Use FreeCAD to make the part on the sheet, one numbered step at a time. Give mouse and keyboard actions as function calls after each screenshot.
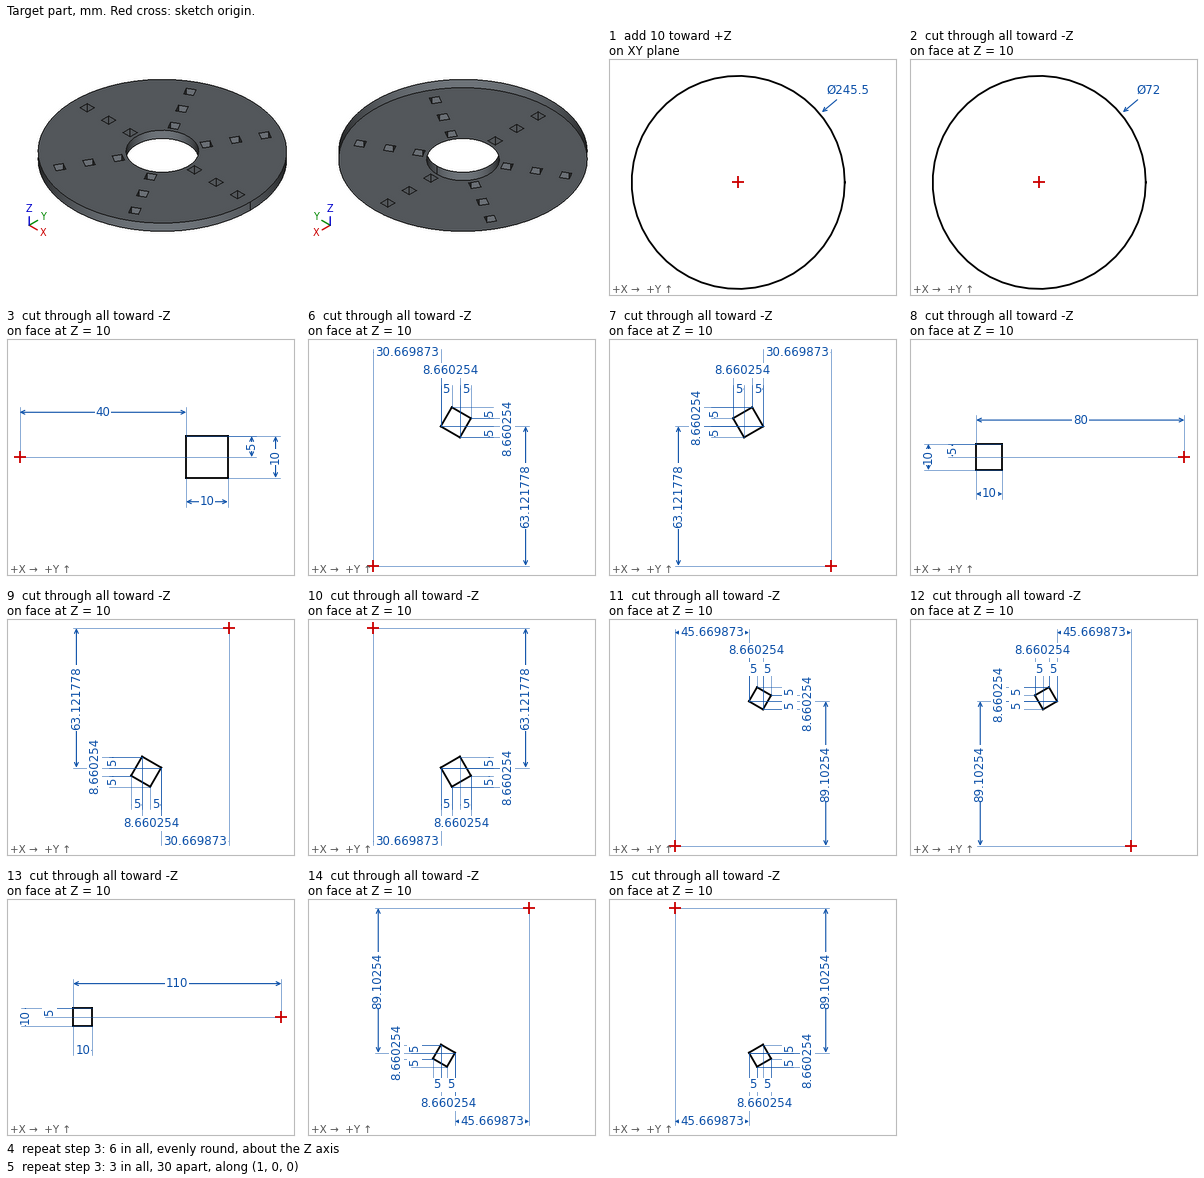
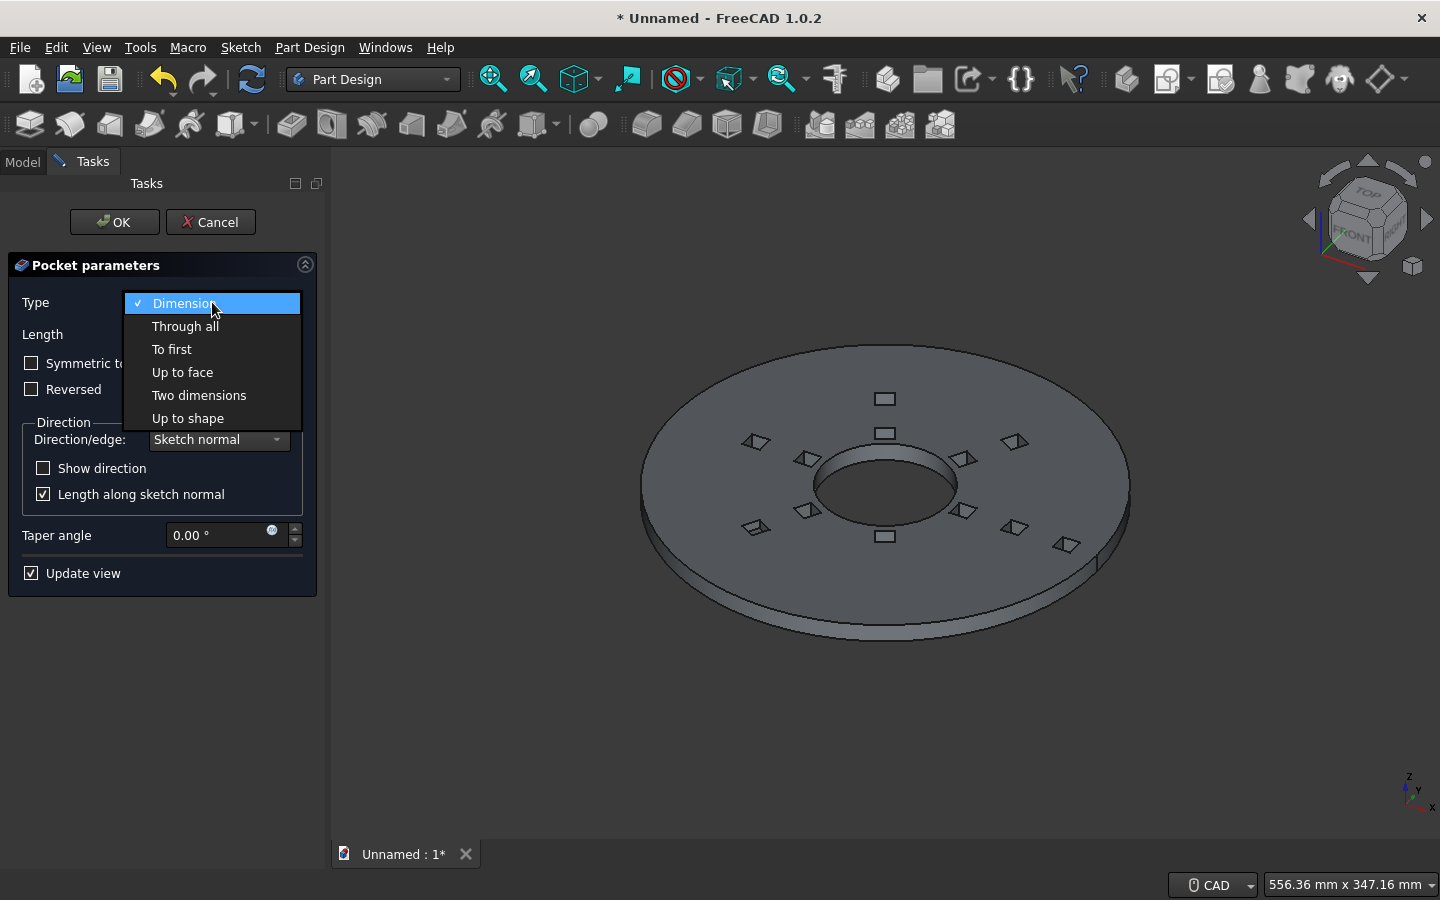
click(212, 326)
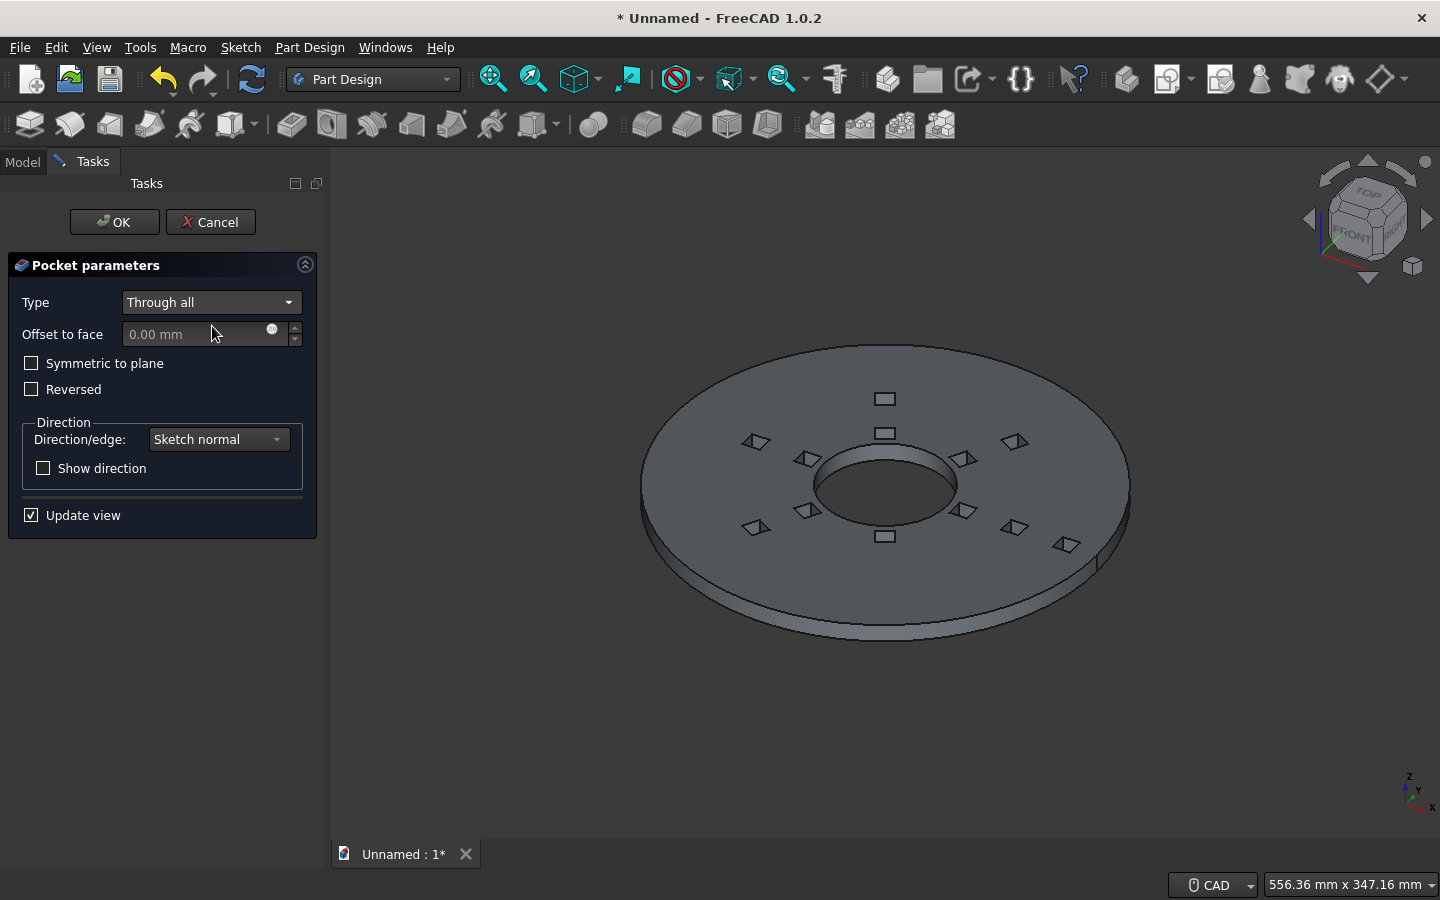
click(115, 222)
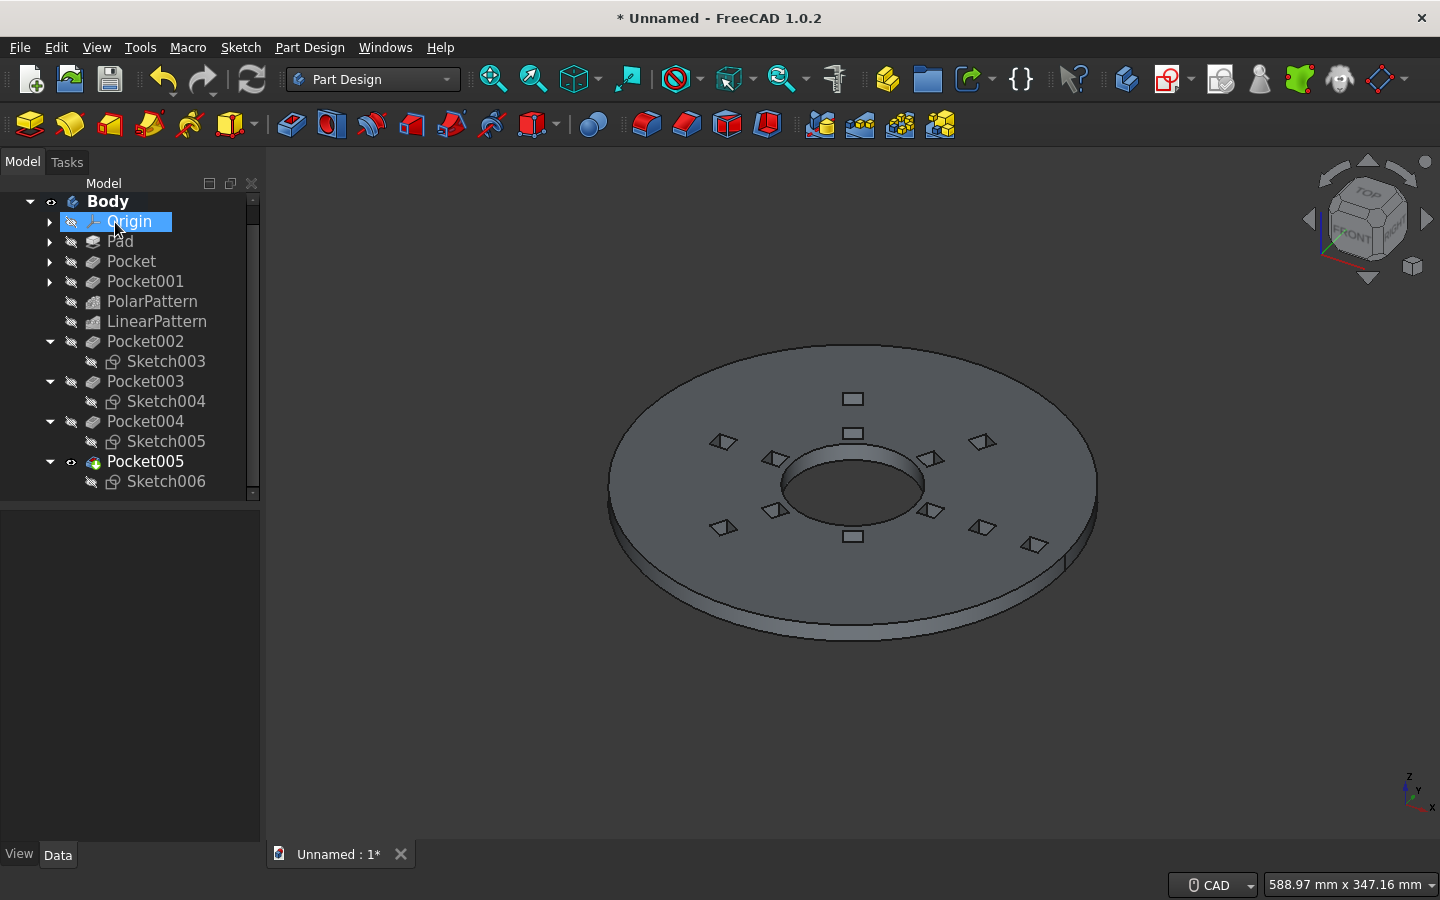
click(923, 414)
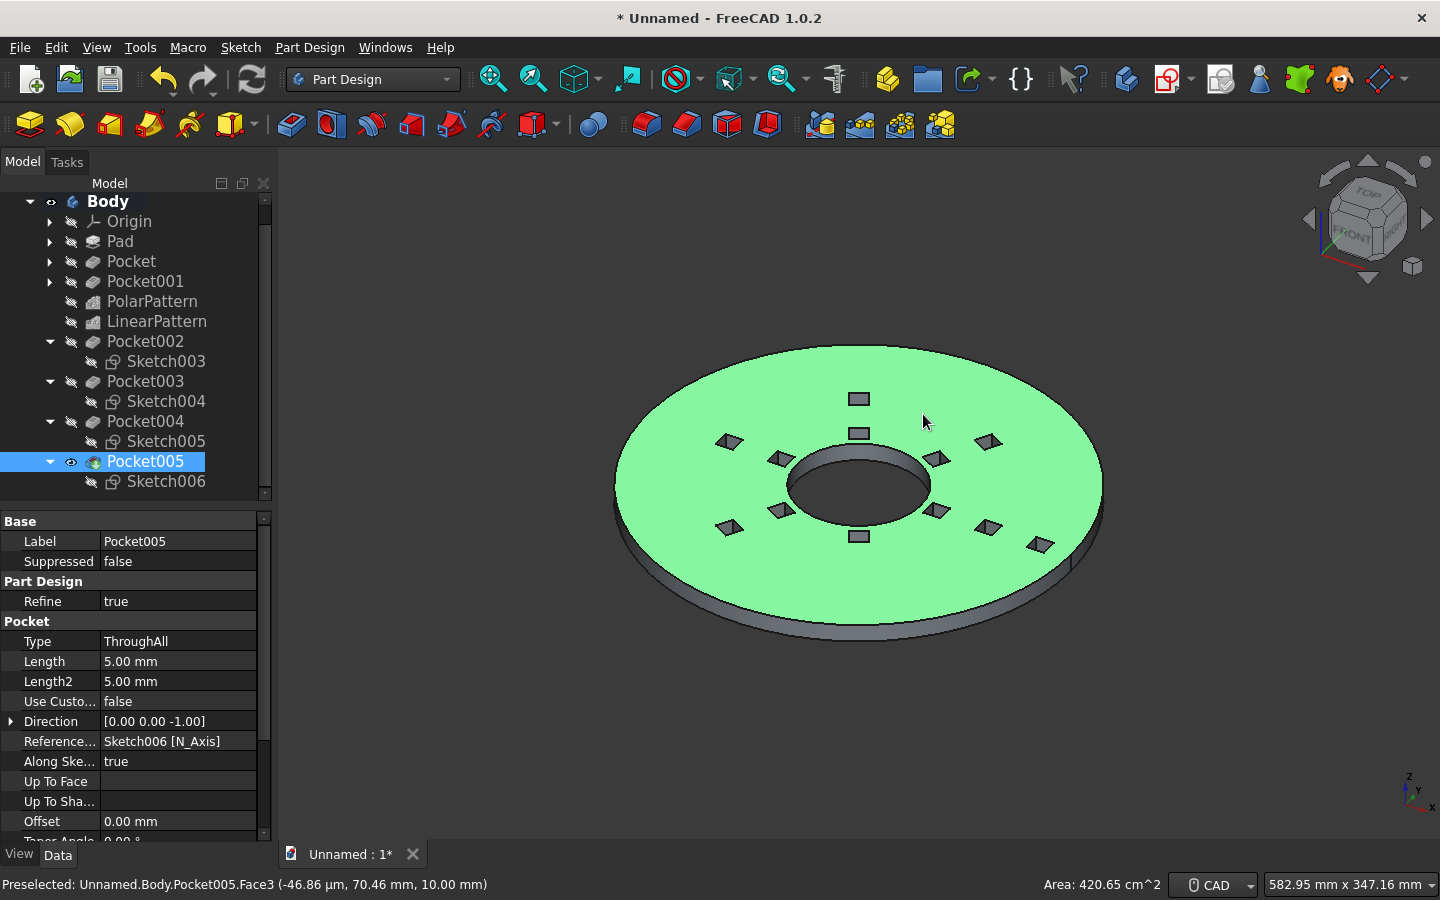
click(1168, 80)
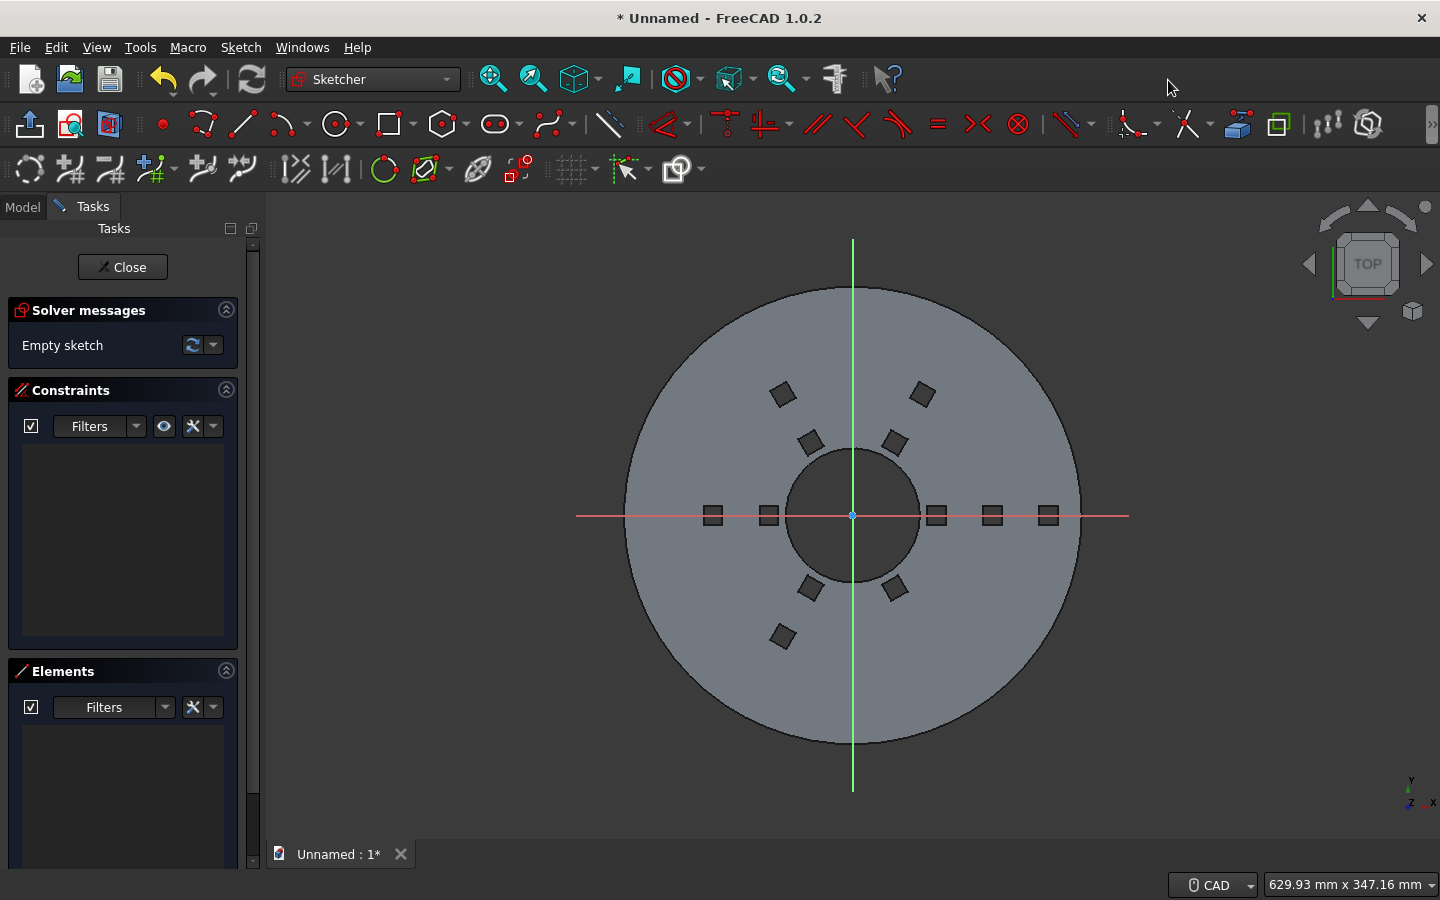
scroll(932, 644, up, 14)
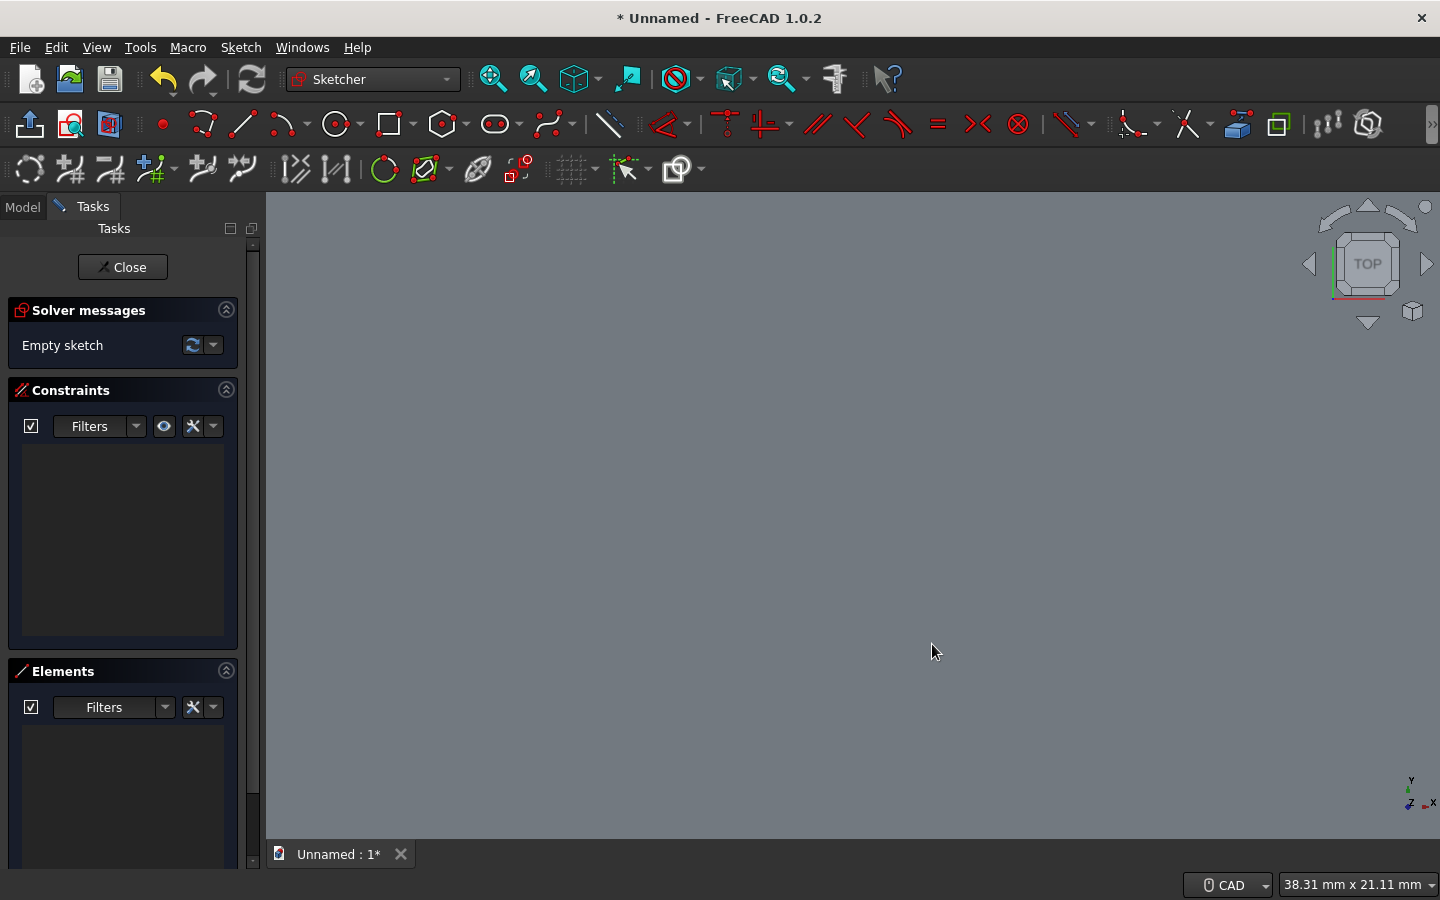
key(g)
key(m)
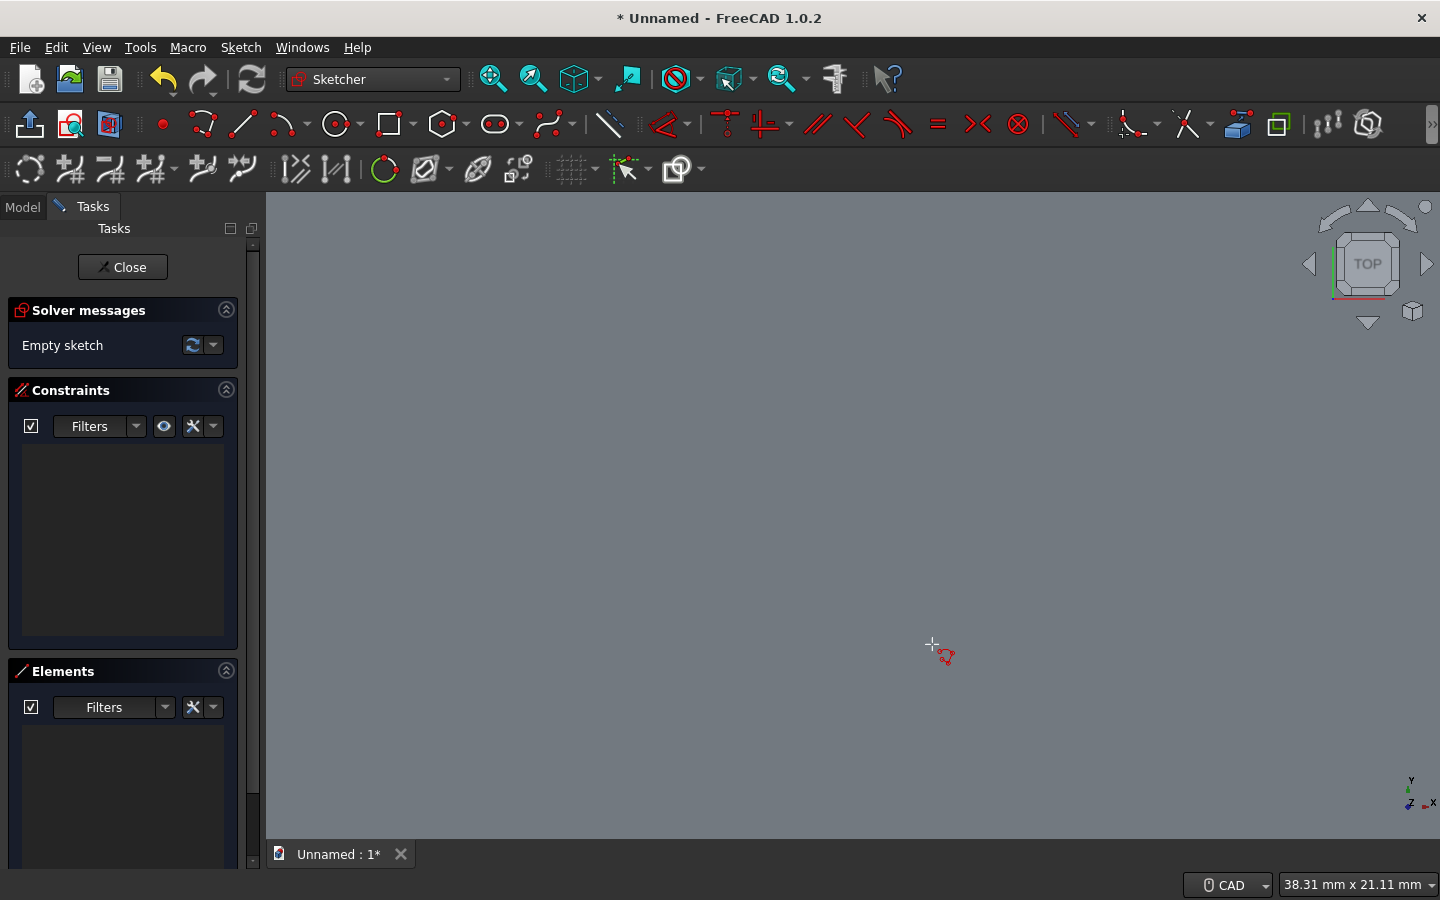
click(562, 455)
click(715, 720)
click(980, 567)
click(827, 301)
click(562, 456)
key(Escape)
key(Escape)